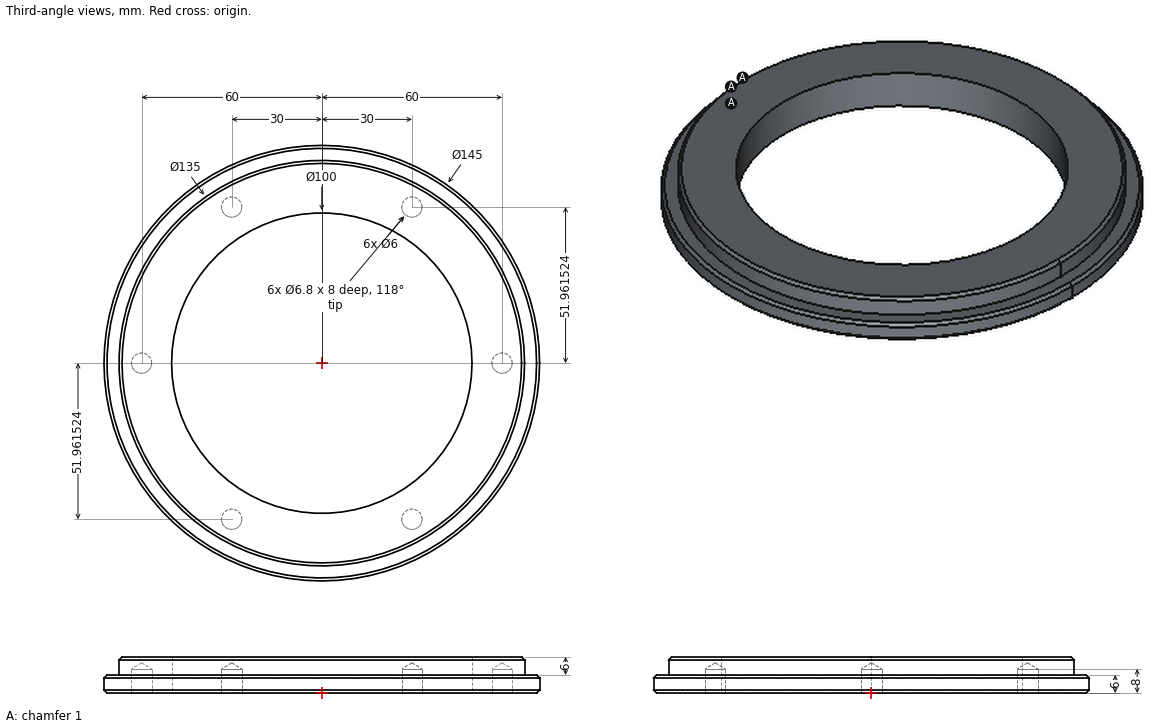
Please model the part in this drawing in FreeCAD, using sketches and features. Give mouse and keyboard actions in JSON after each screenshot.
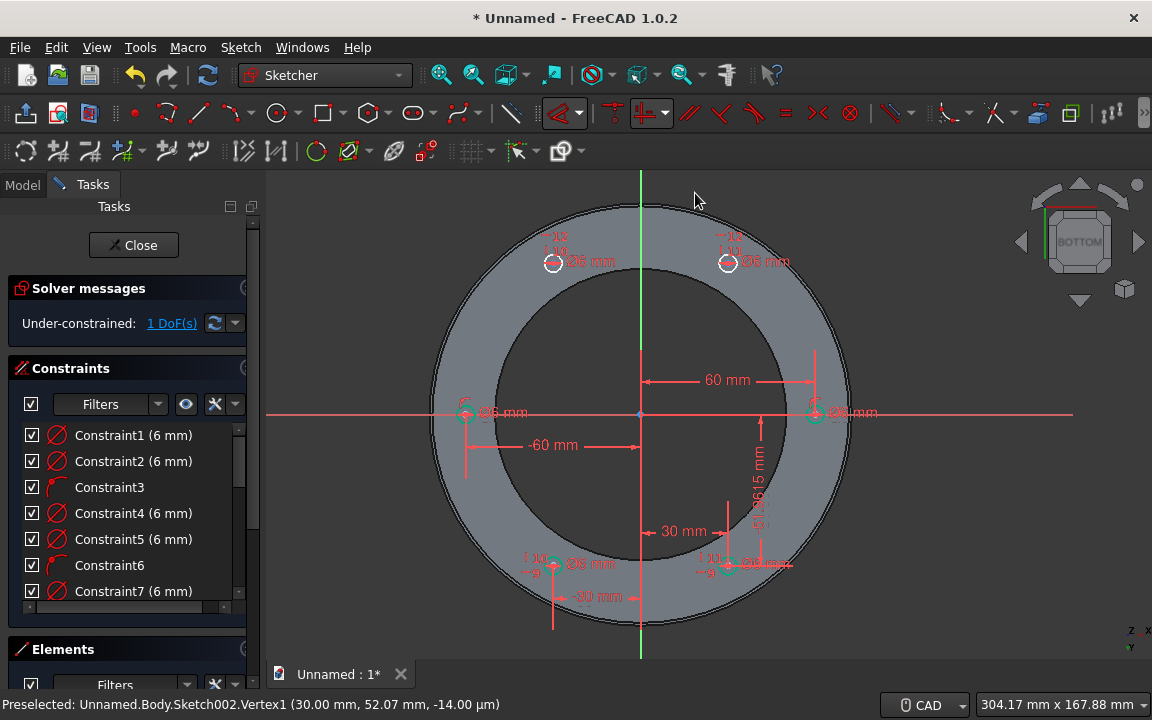
{"action": "left_click", "coordinate": [553, 263]}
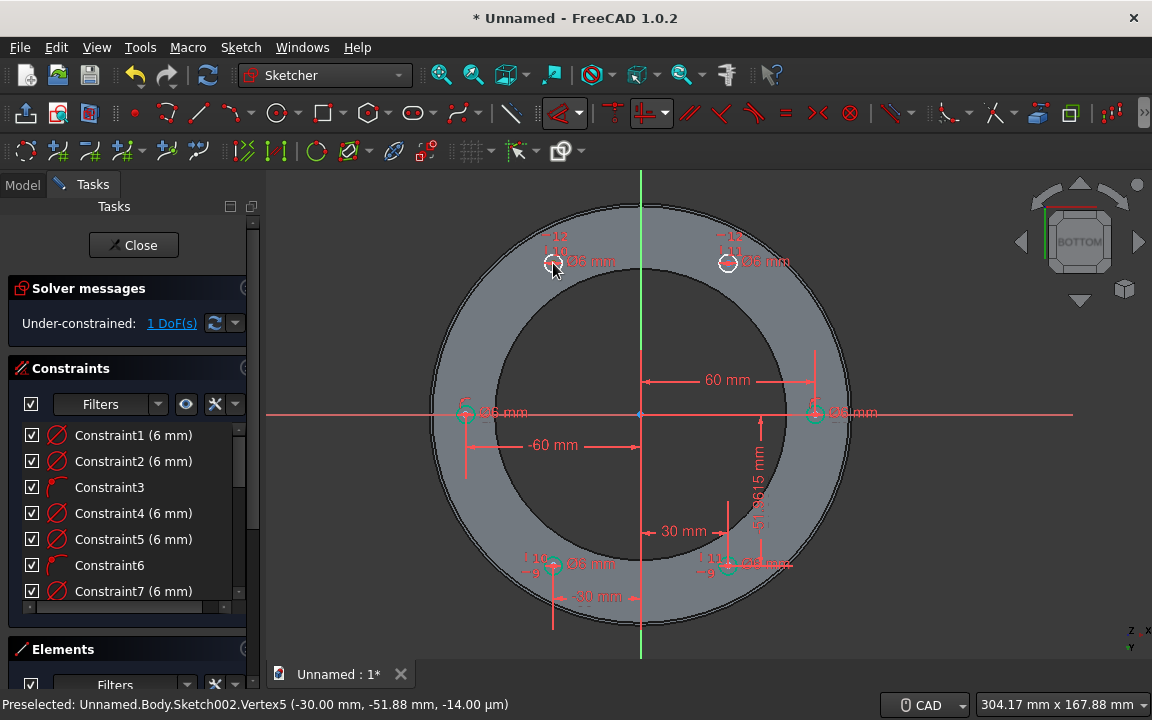
{"action": "left_click", "coordinate": [582, 114]}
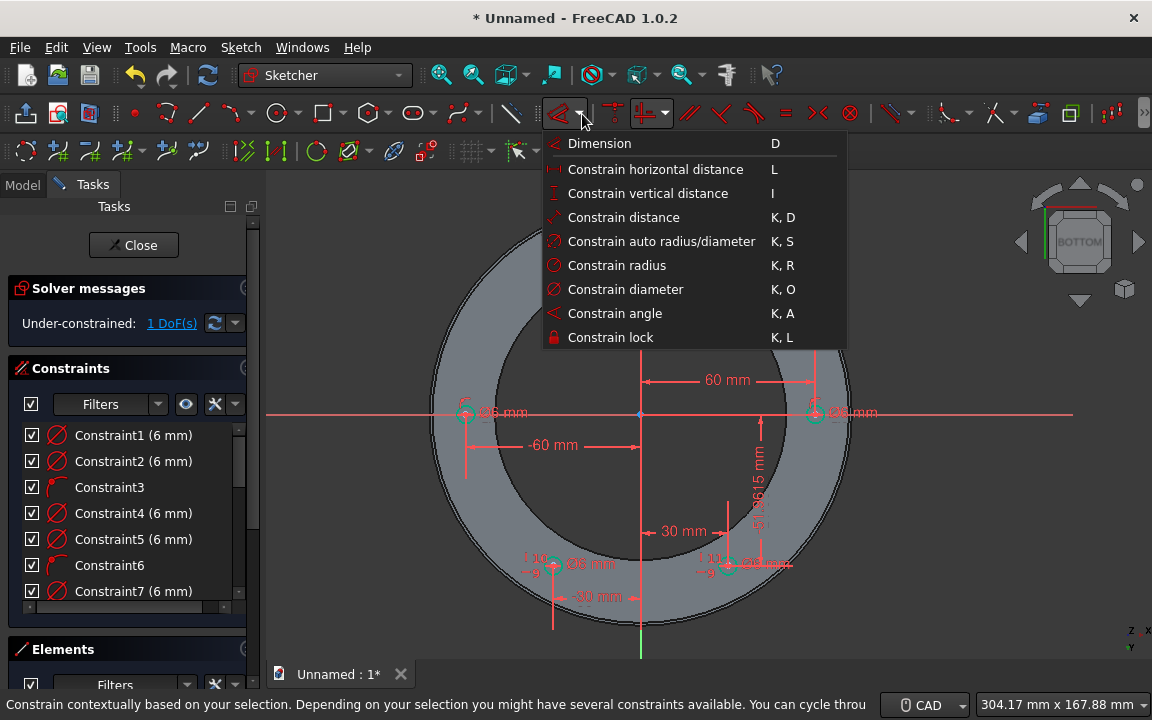
{"action": "left_click", "coordinate": [695, 193]}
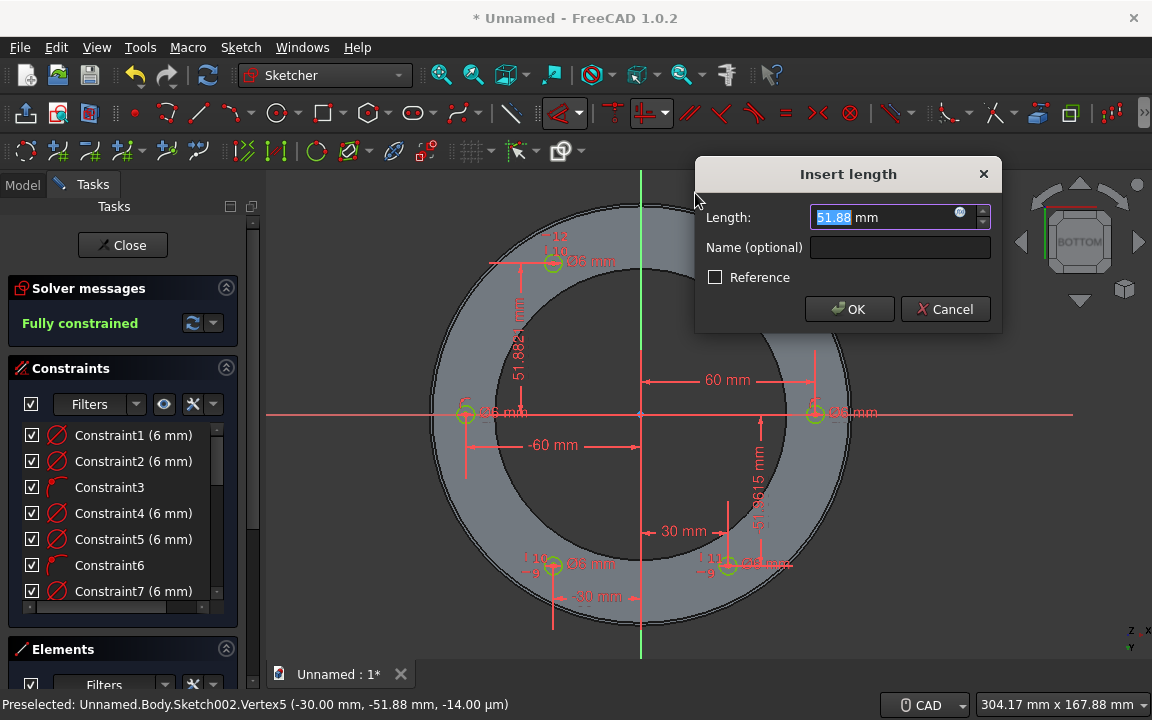
{"action": "type", "text": "51.961524"}
{"action": "key", "text": "Return"}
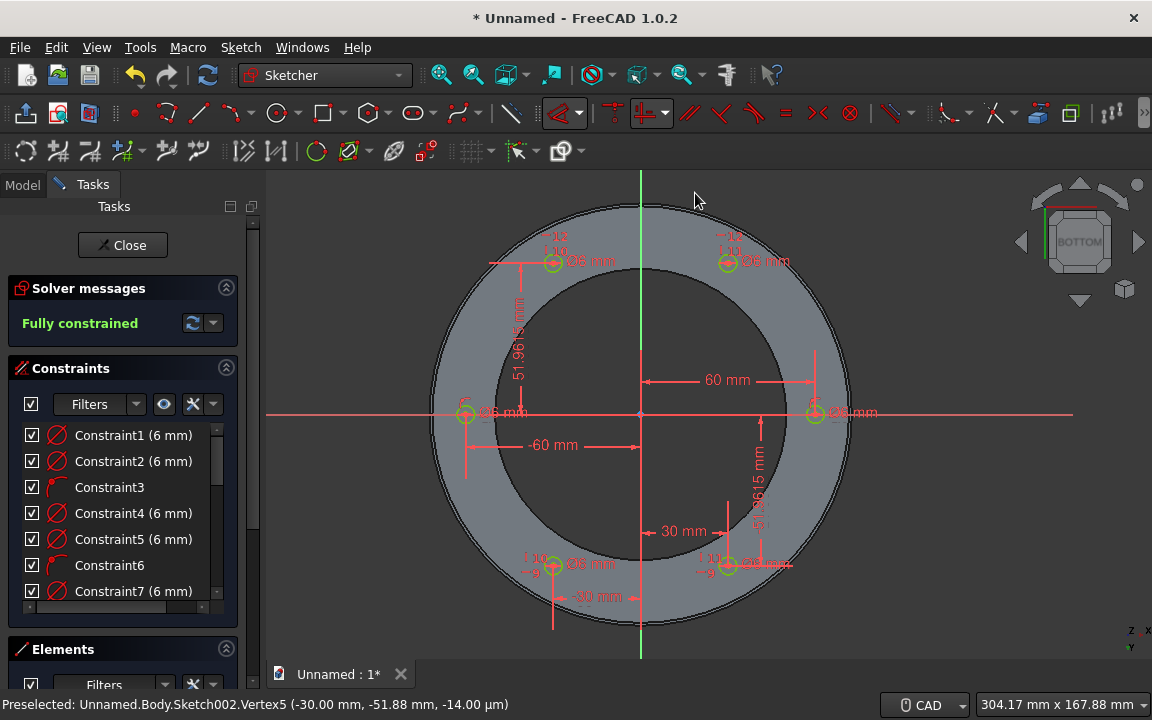
{"action": "left_click", "coordinate": [123, 245]}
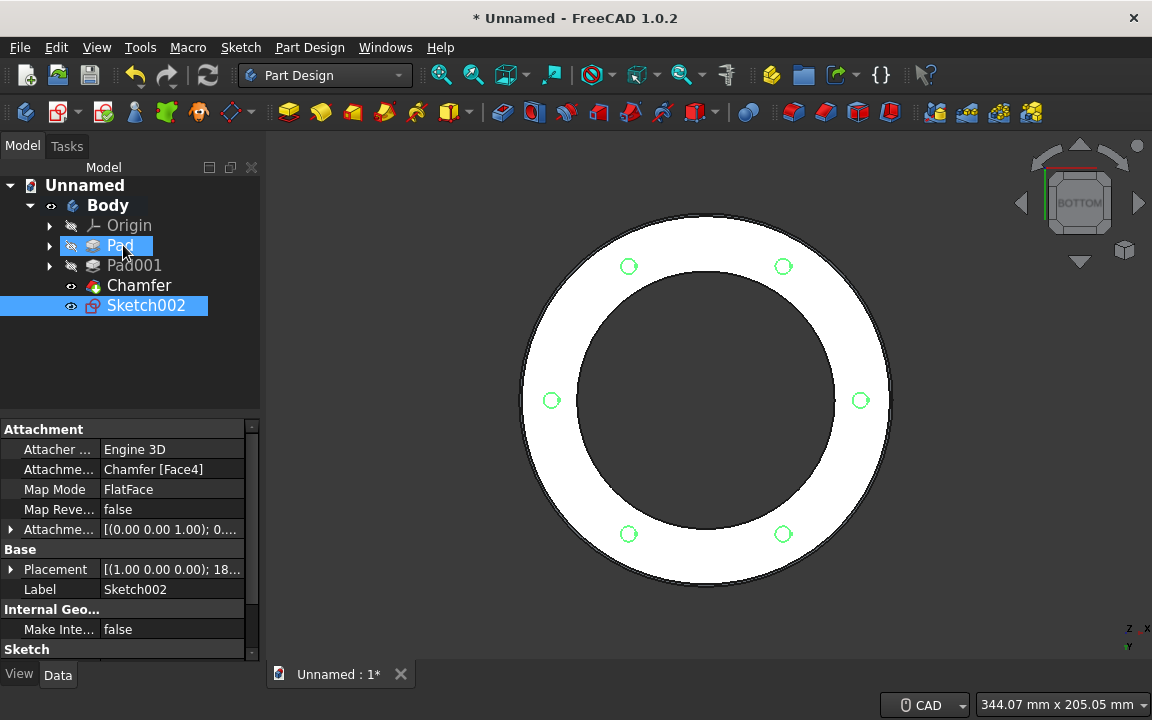
{"action": "left_click", "coordinate": [504, 112]}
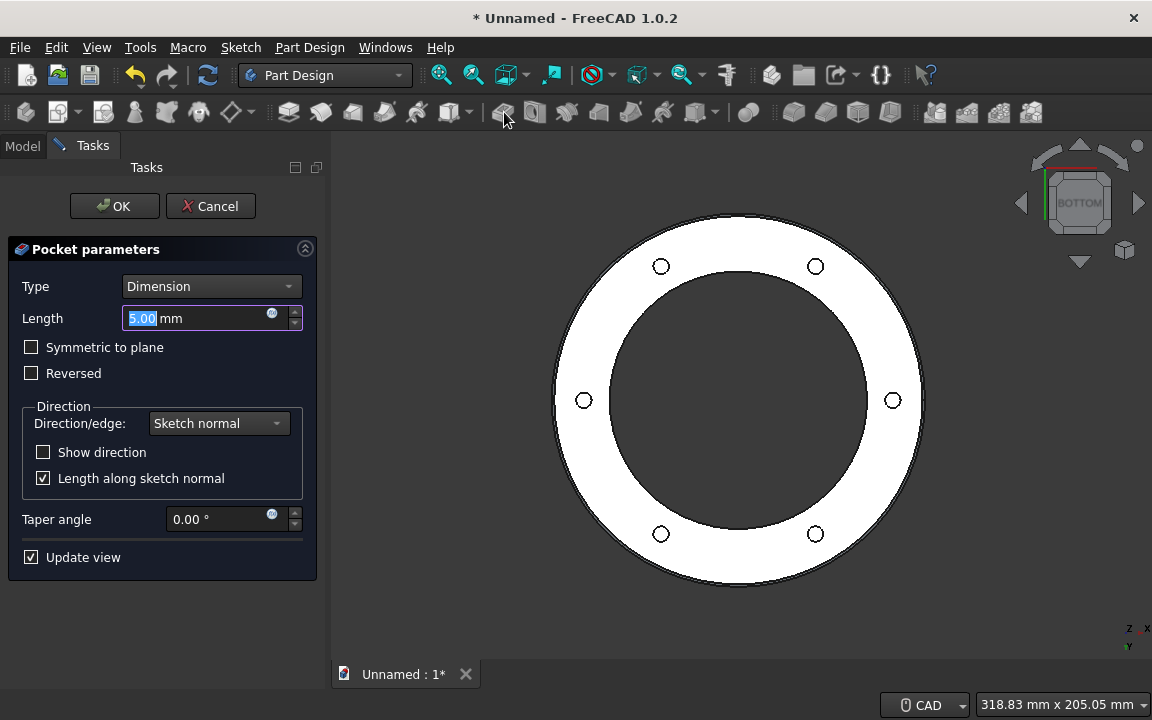
{"action": "type", "text": "8"}
{"action": "key", "text": "Tab"}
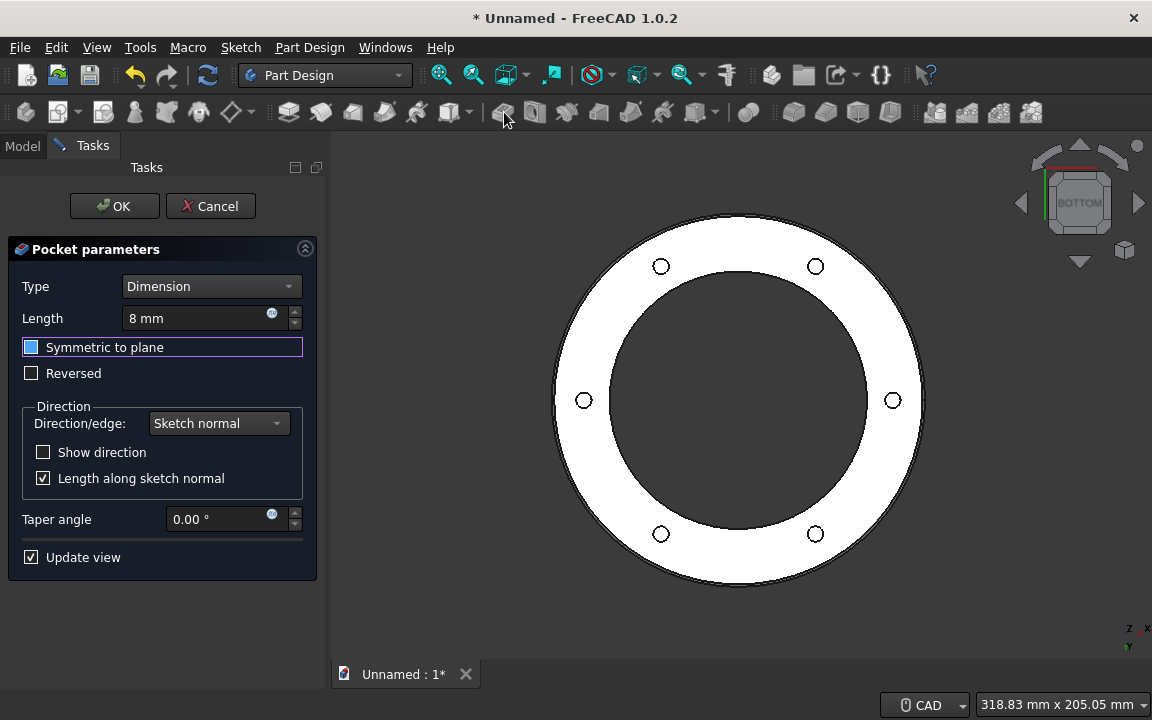
{"action": "left_click", "coordinate": [115, 206]}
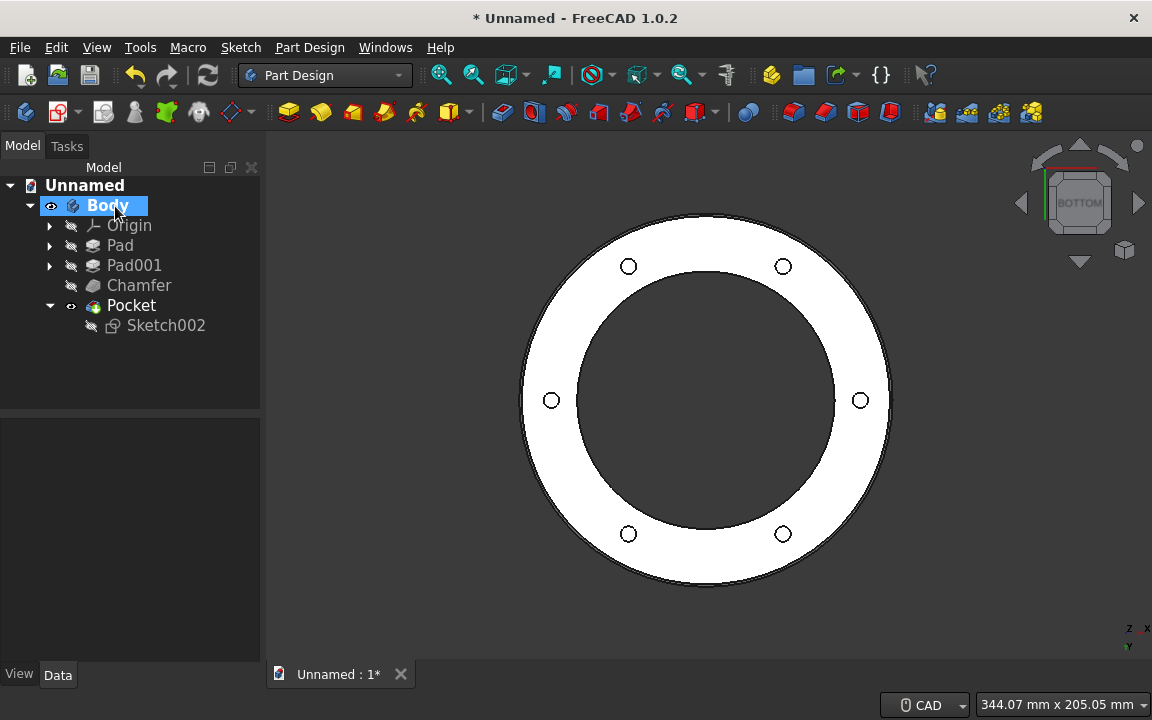
{"action": "left_click", "coordinate": [58, 112]}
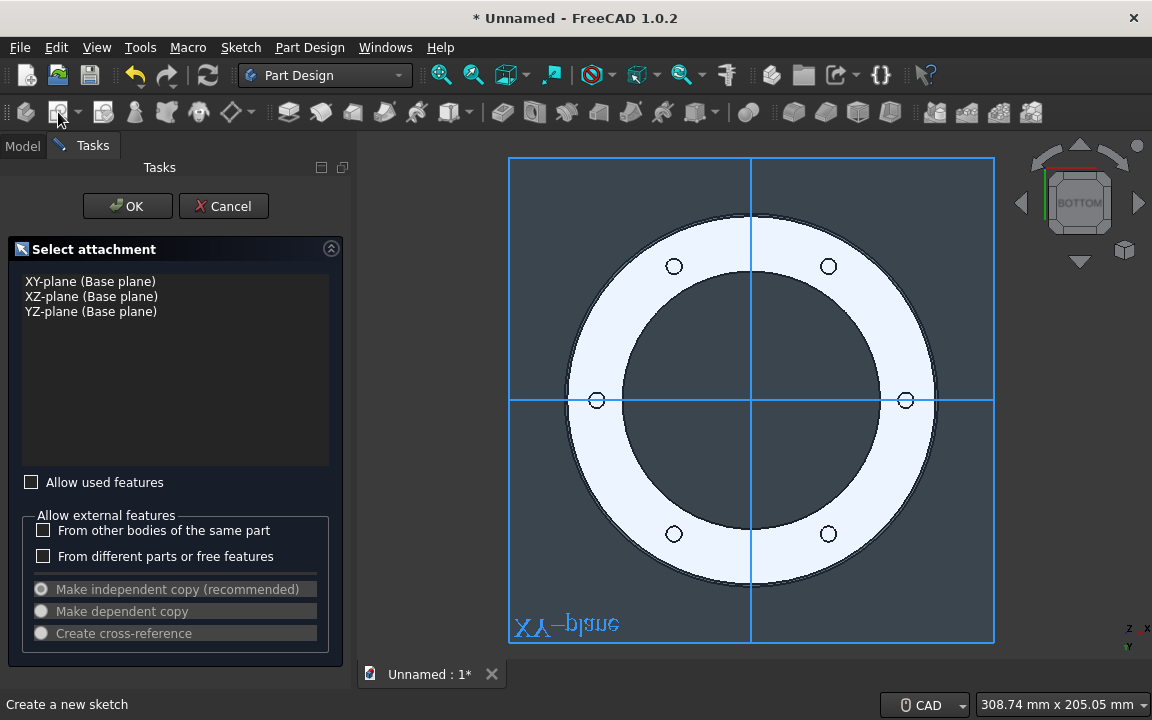
{"action": "left_click", "coordinate": [82, 282]}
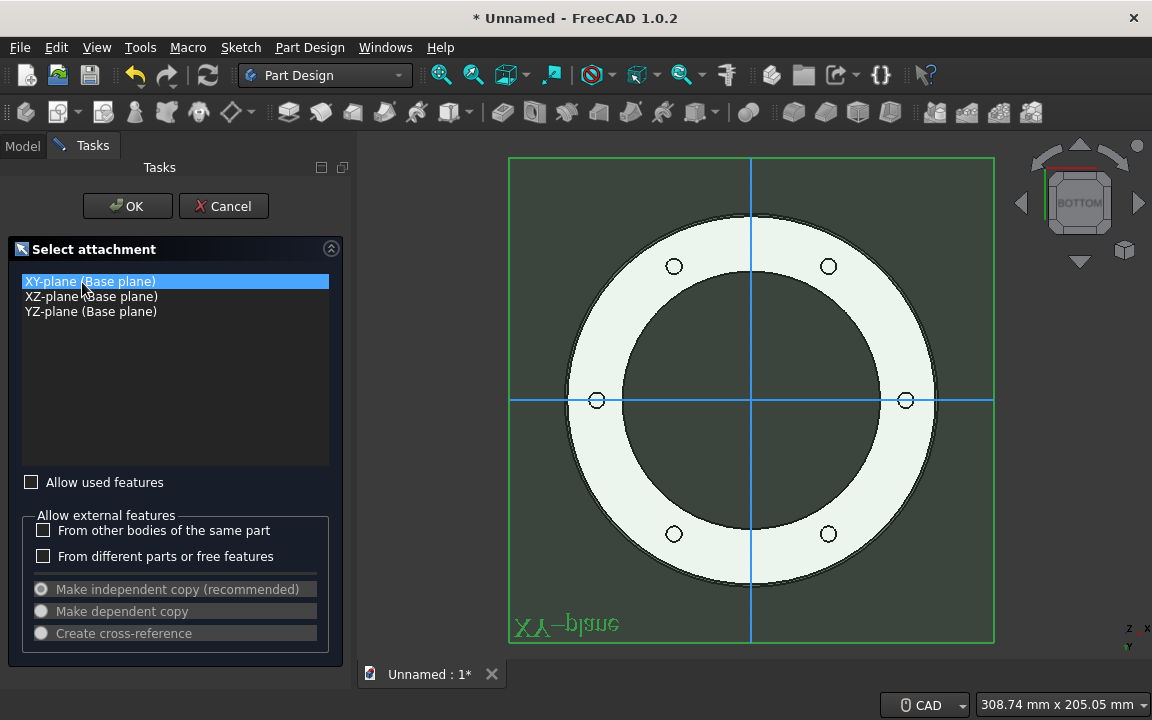
{"action": "left_click", "coordinate": [128, 206]}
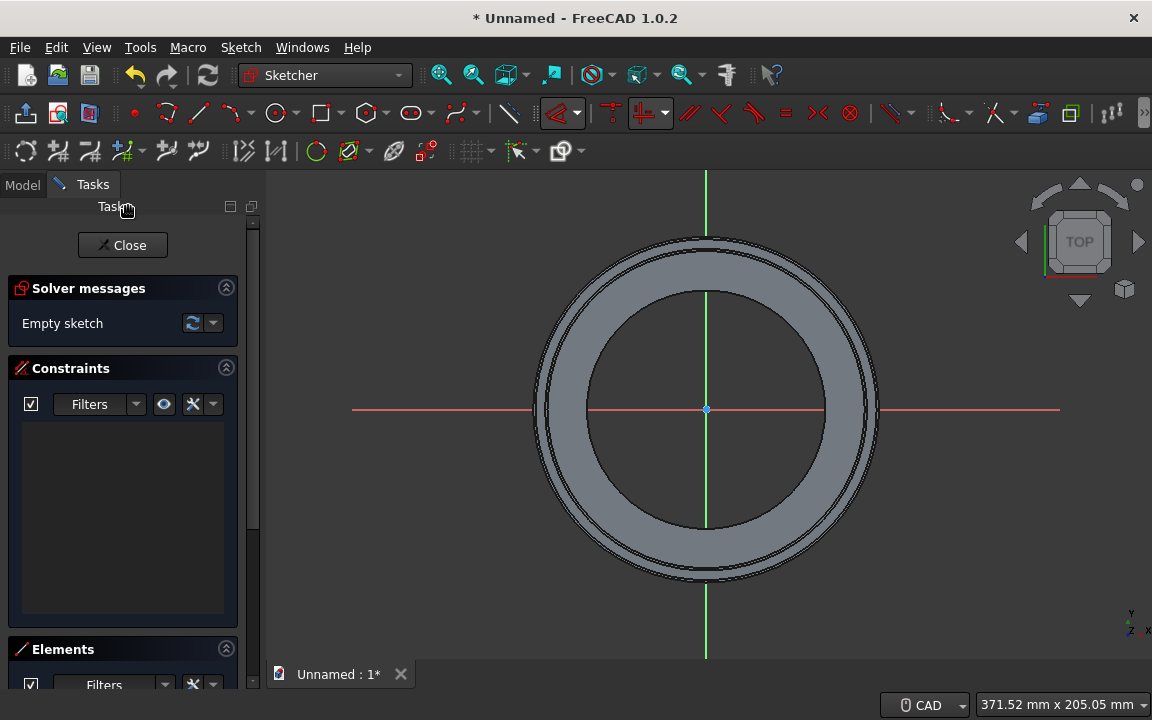
{"action": "left_click", "coordinate": [90, 114]}